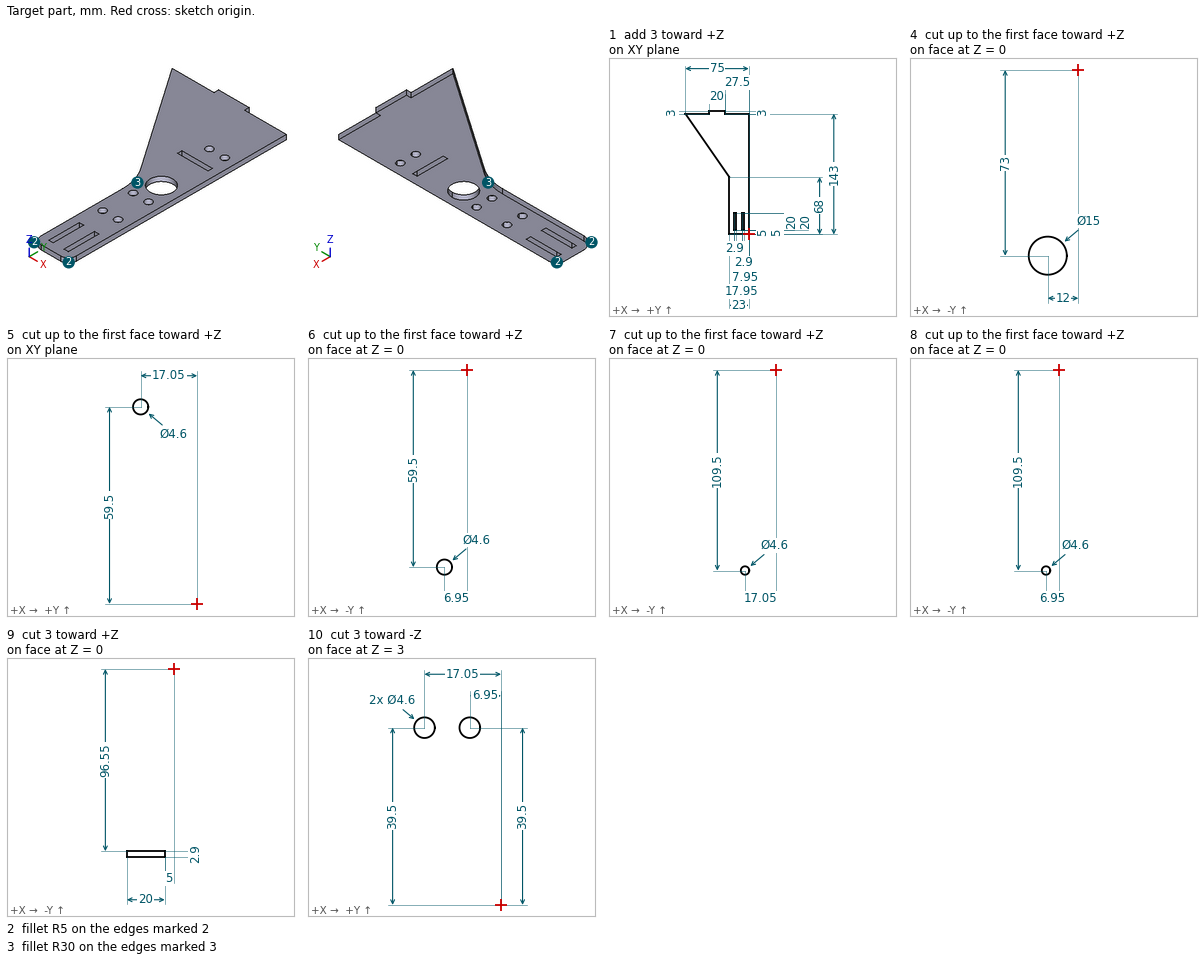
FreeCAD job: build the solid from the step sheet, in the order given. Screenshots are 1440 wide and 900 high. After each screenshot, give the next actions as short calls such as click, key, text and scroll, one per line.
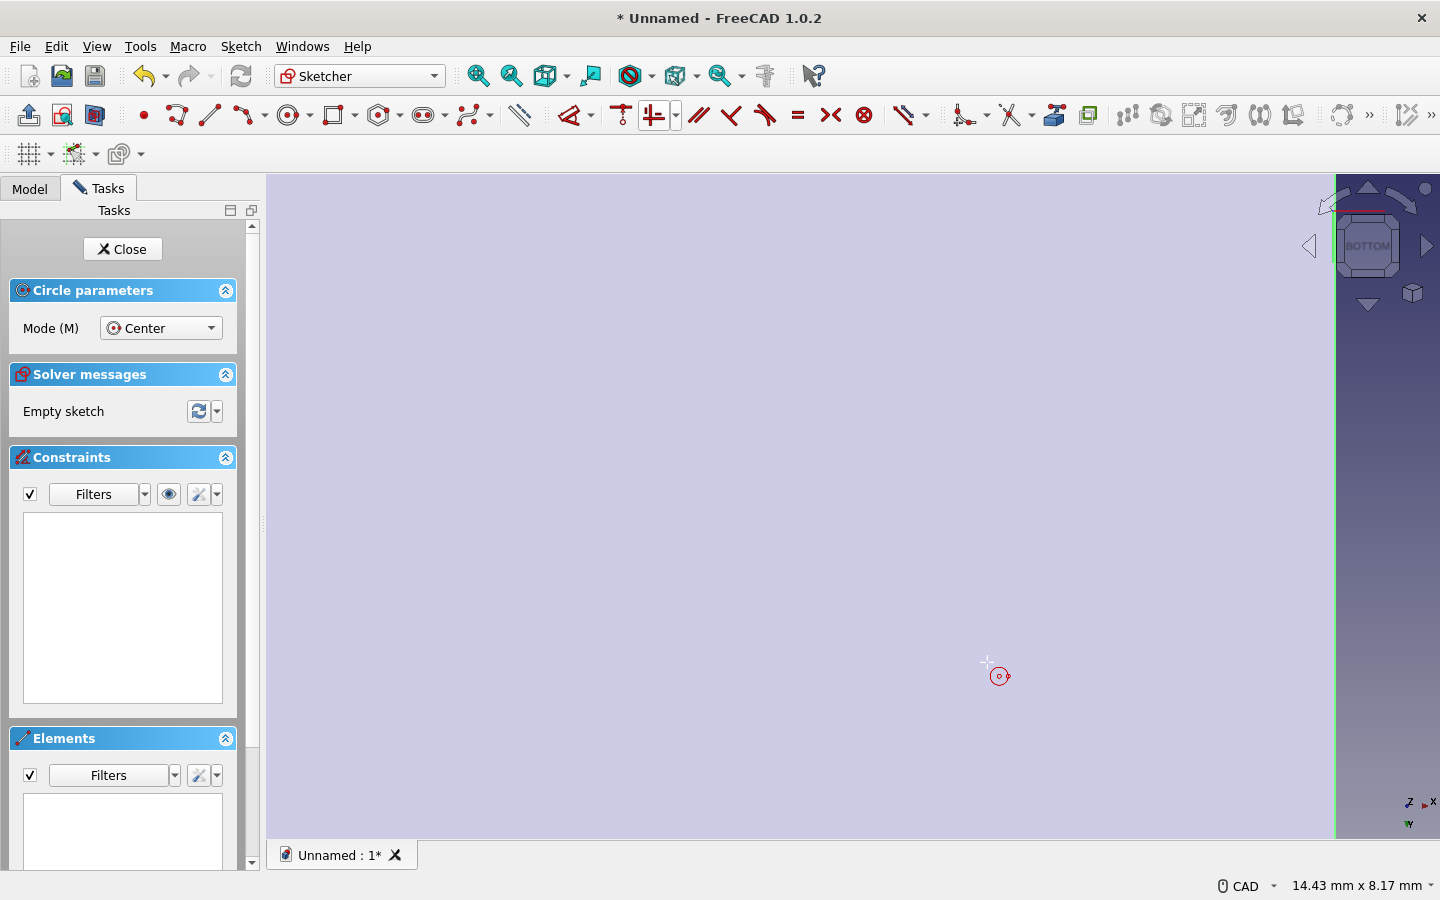
click(769, 494)
move(902, 362)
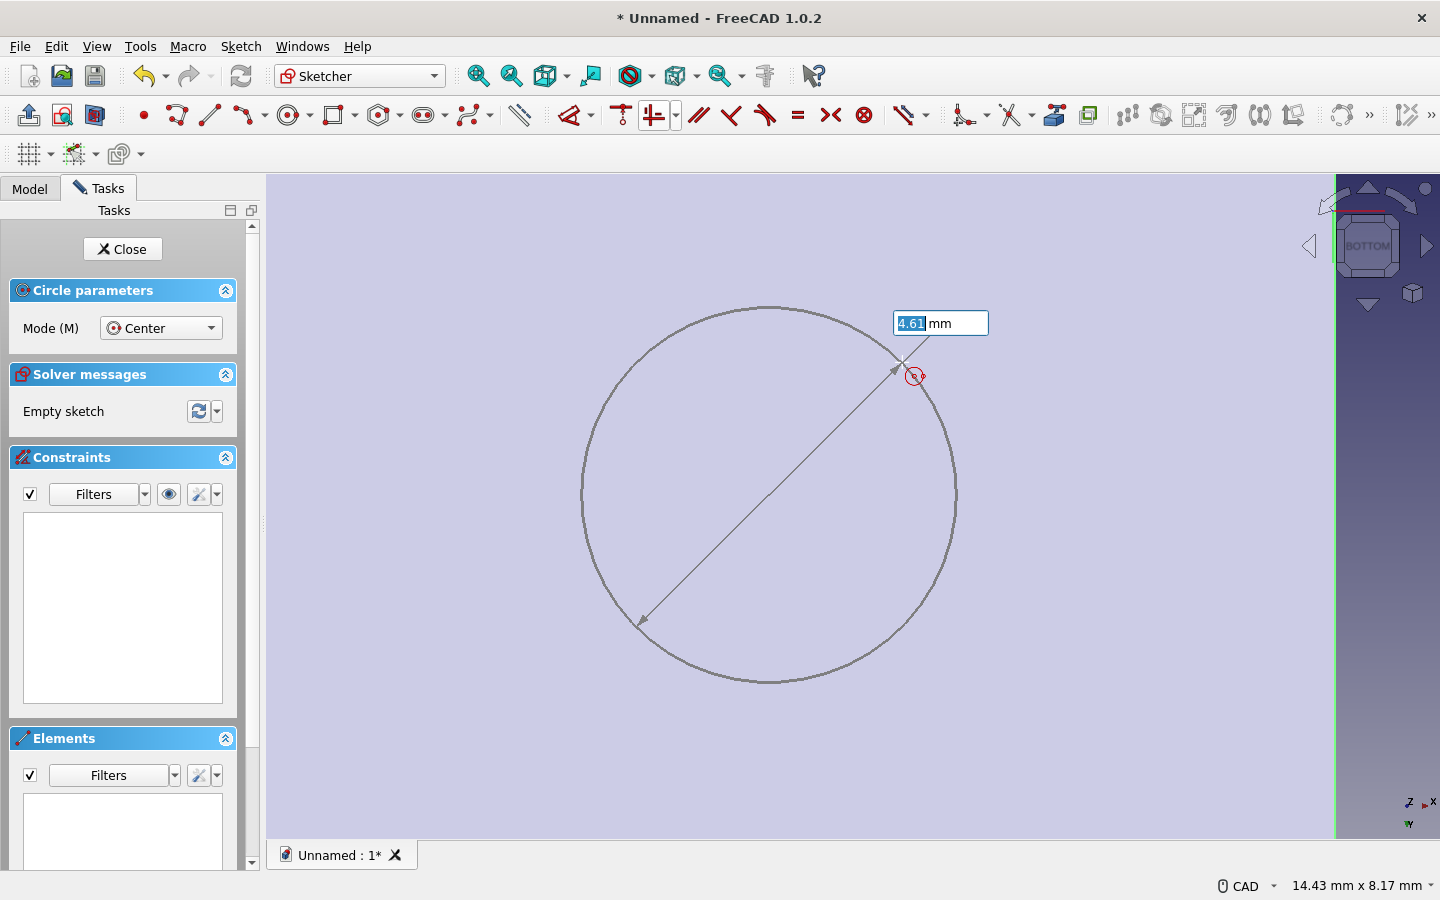
text(4.6)
key(Return)
key(Escape)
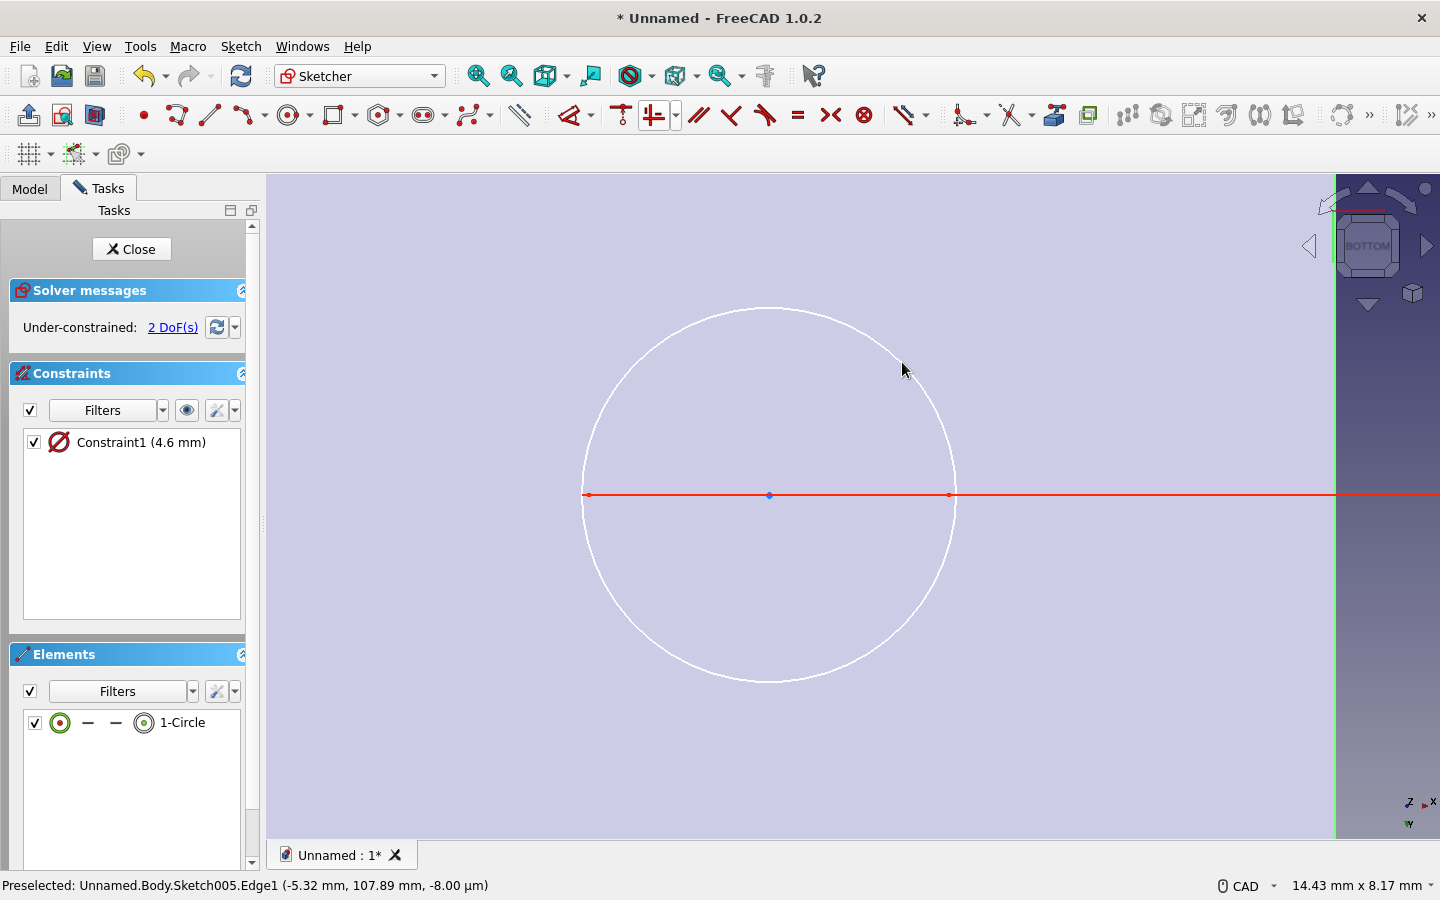
key(d)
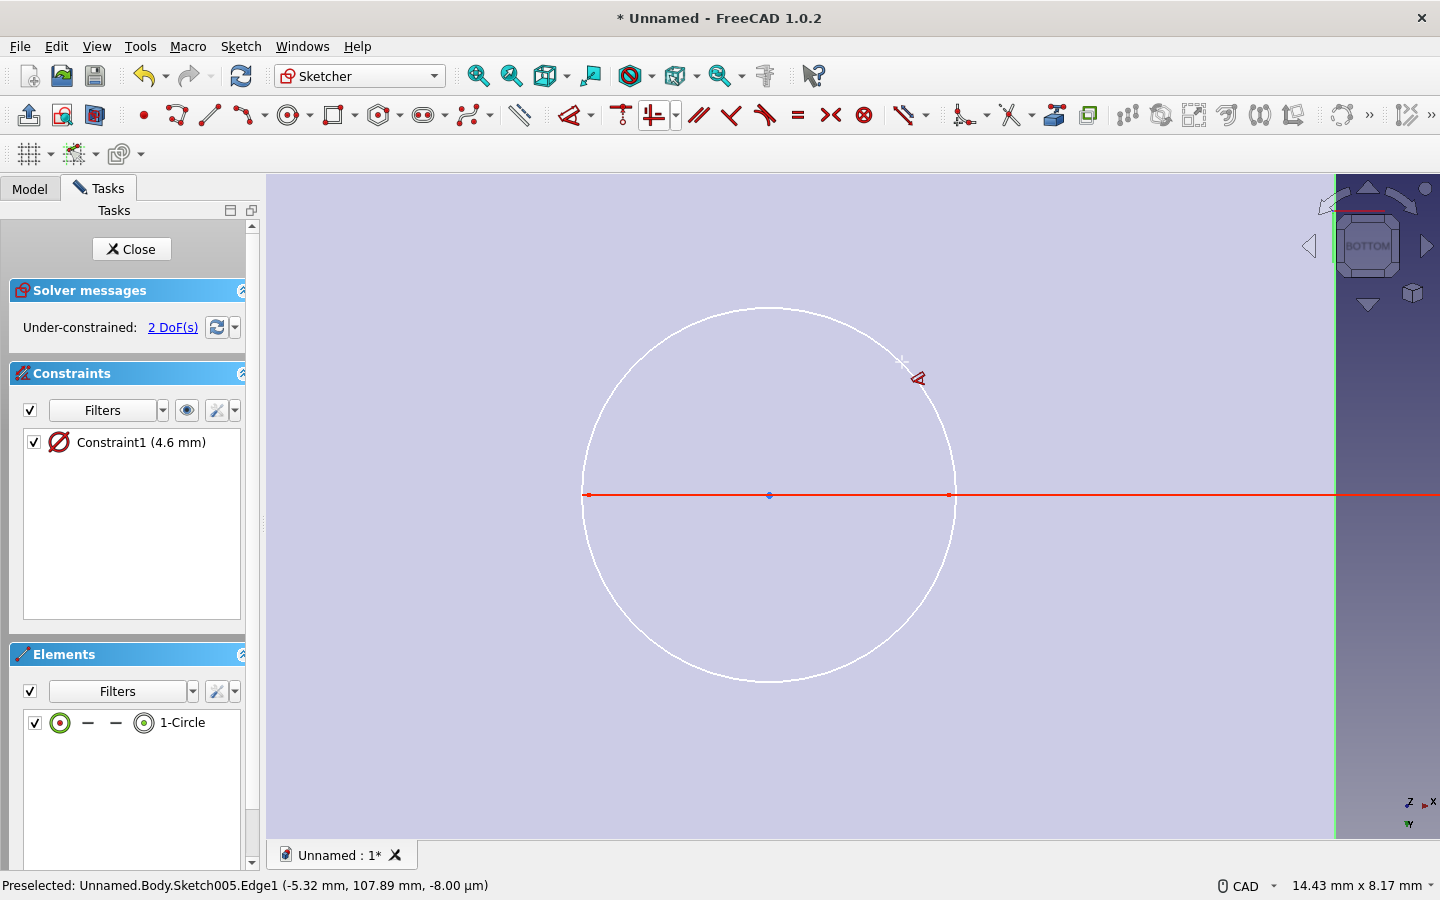
click(769, 495)
click(1022, 529)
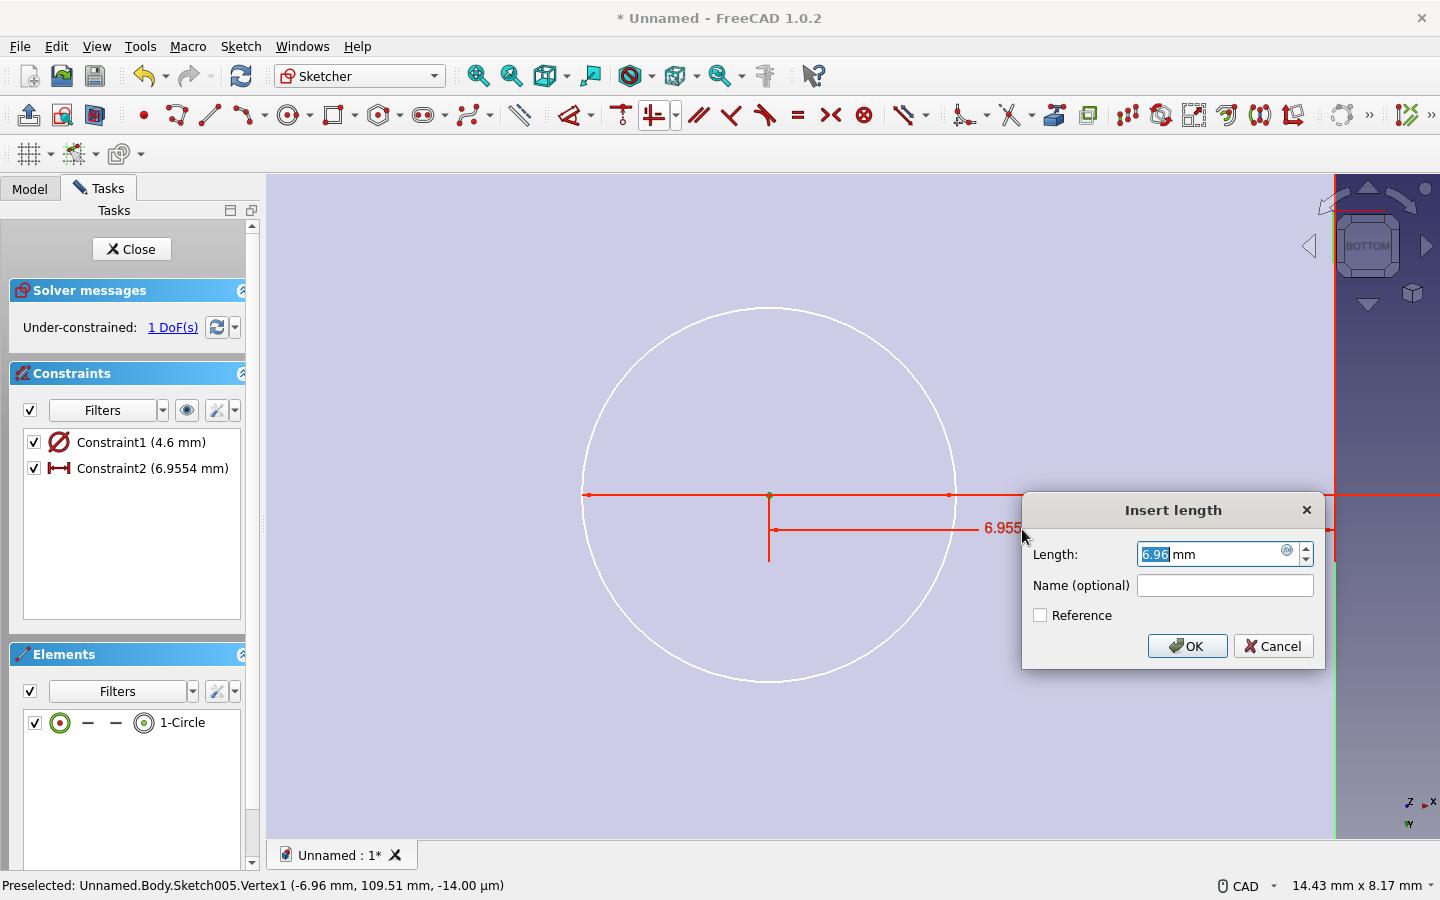
text(6.95)
key(Return)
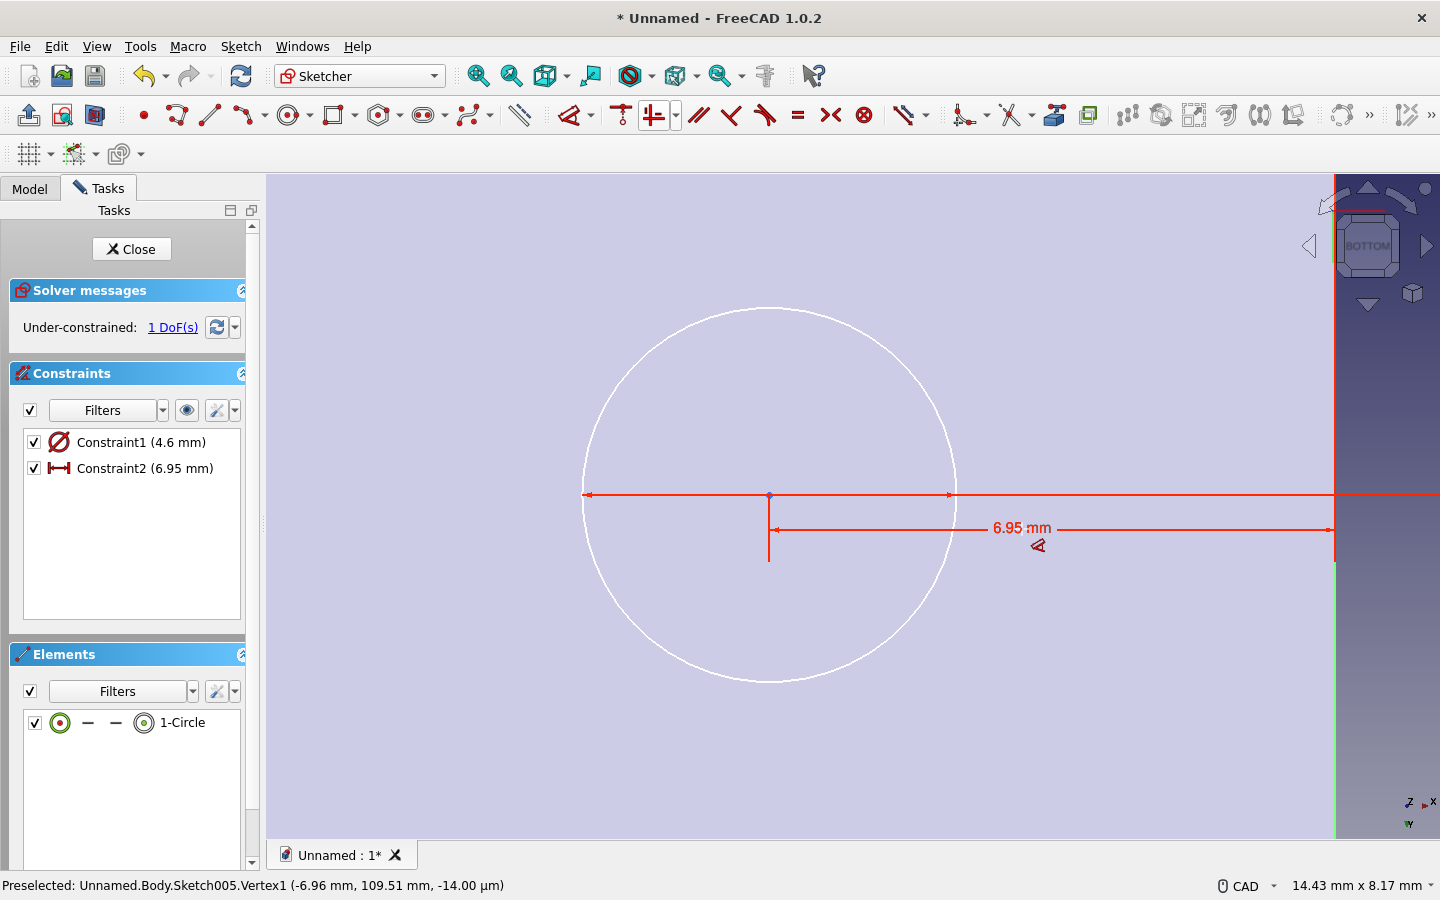
click(769, 495)
click(735, 349)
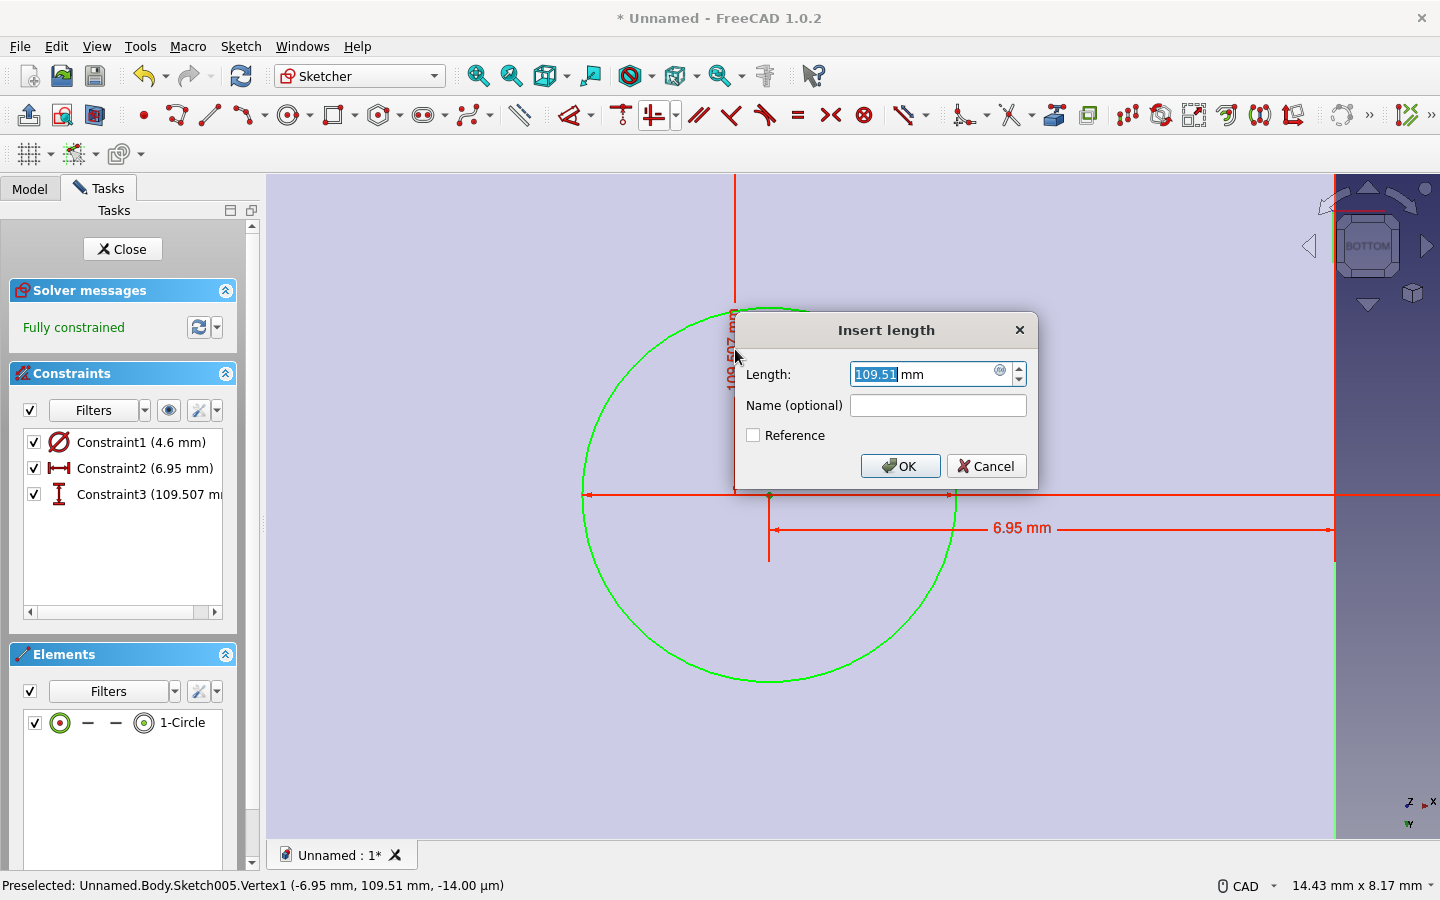
text(109.5)
key(Return)
key(Escape)